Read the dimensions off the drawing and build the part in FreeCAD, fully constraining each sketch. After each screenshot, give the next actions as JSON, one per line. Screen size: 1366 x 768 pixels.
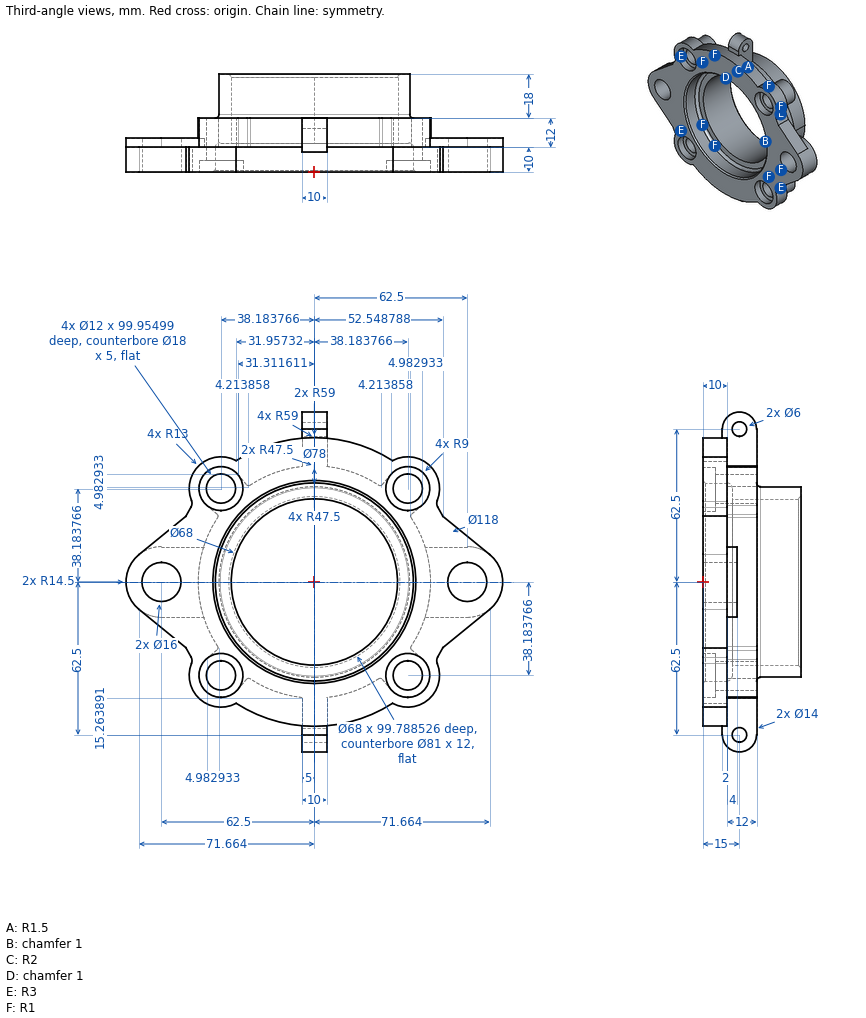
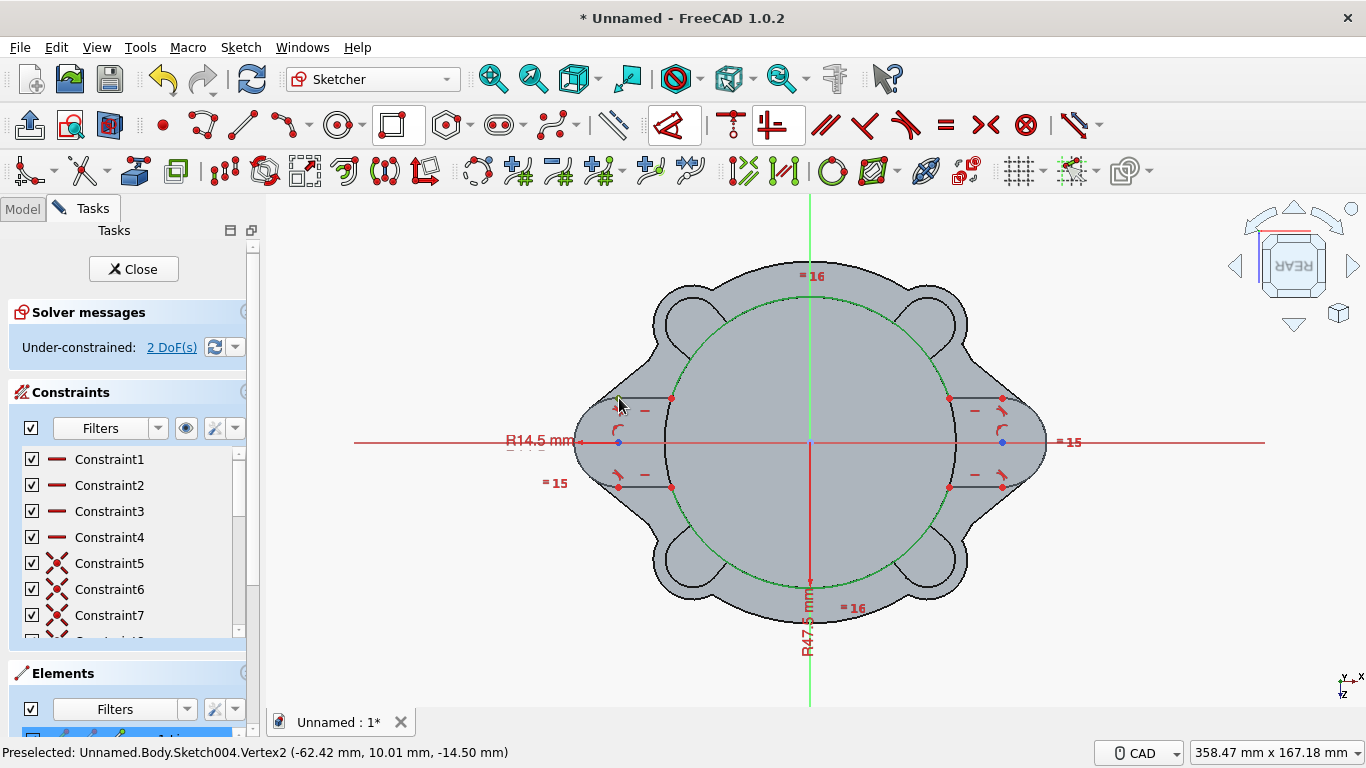
{"action": "key", "text": "l"}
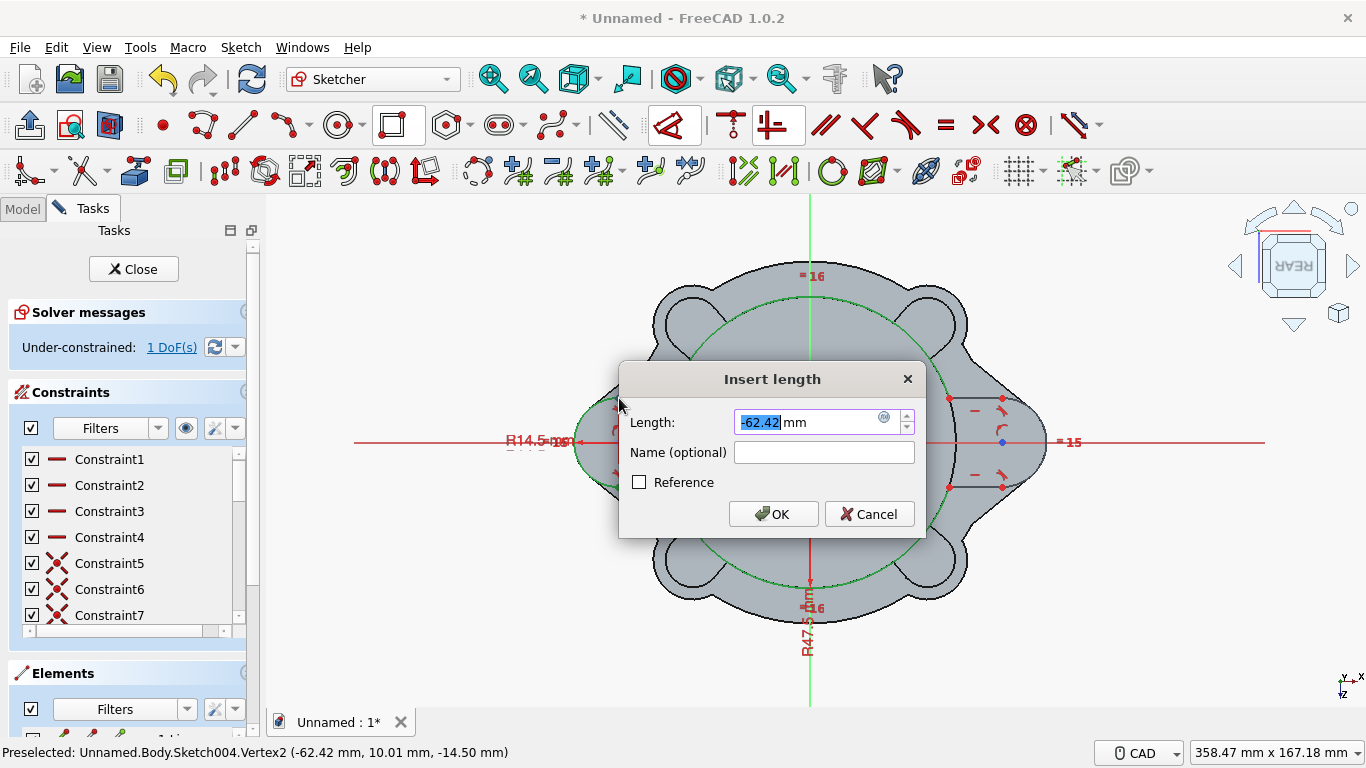
{"action": "type", "text": "-62.5"}
{"action": "key", "text": "Return"}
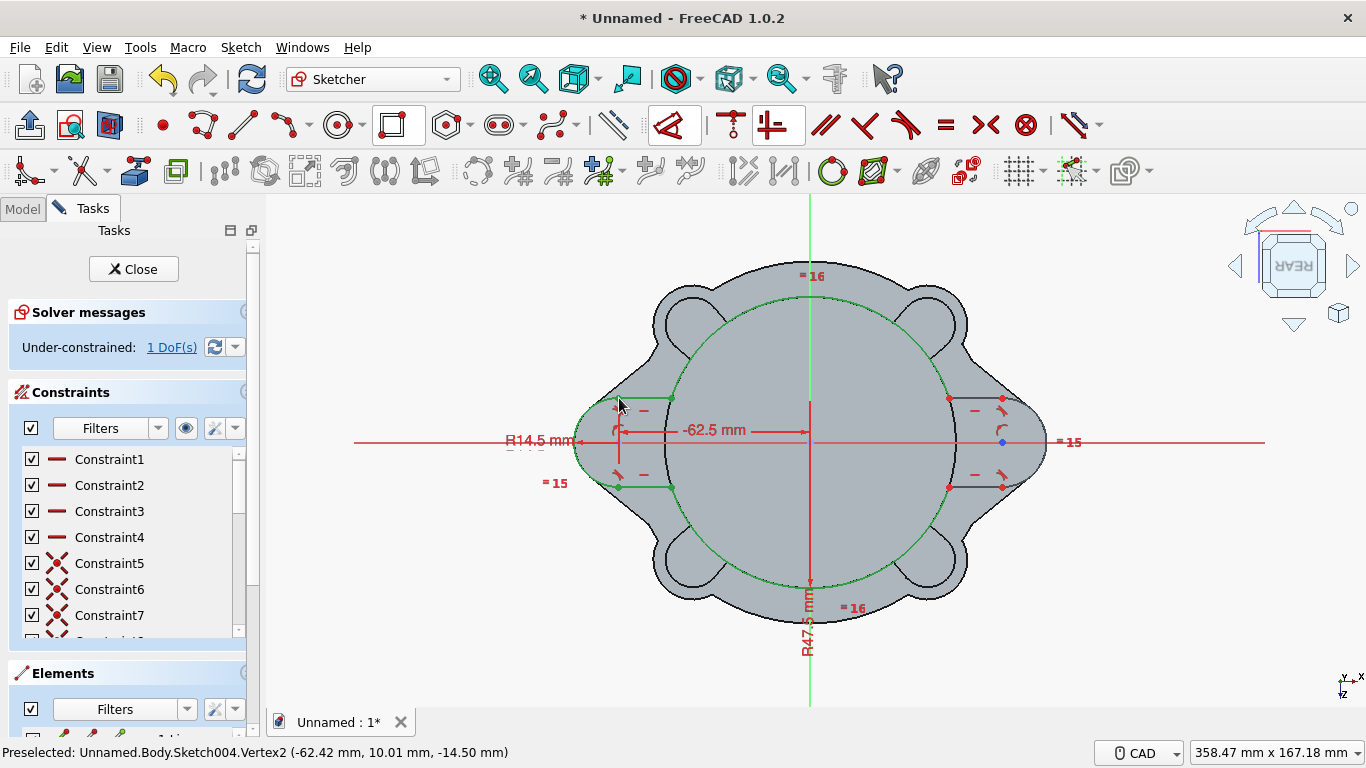
{"action": "left_click", "coordinate": [1002, 487]}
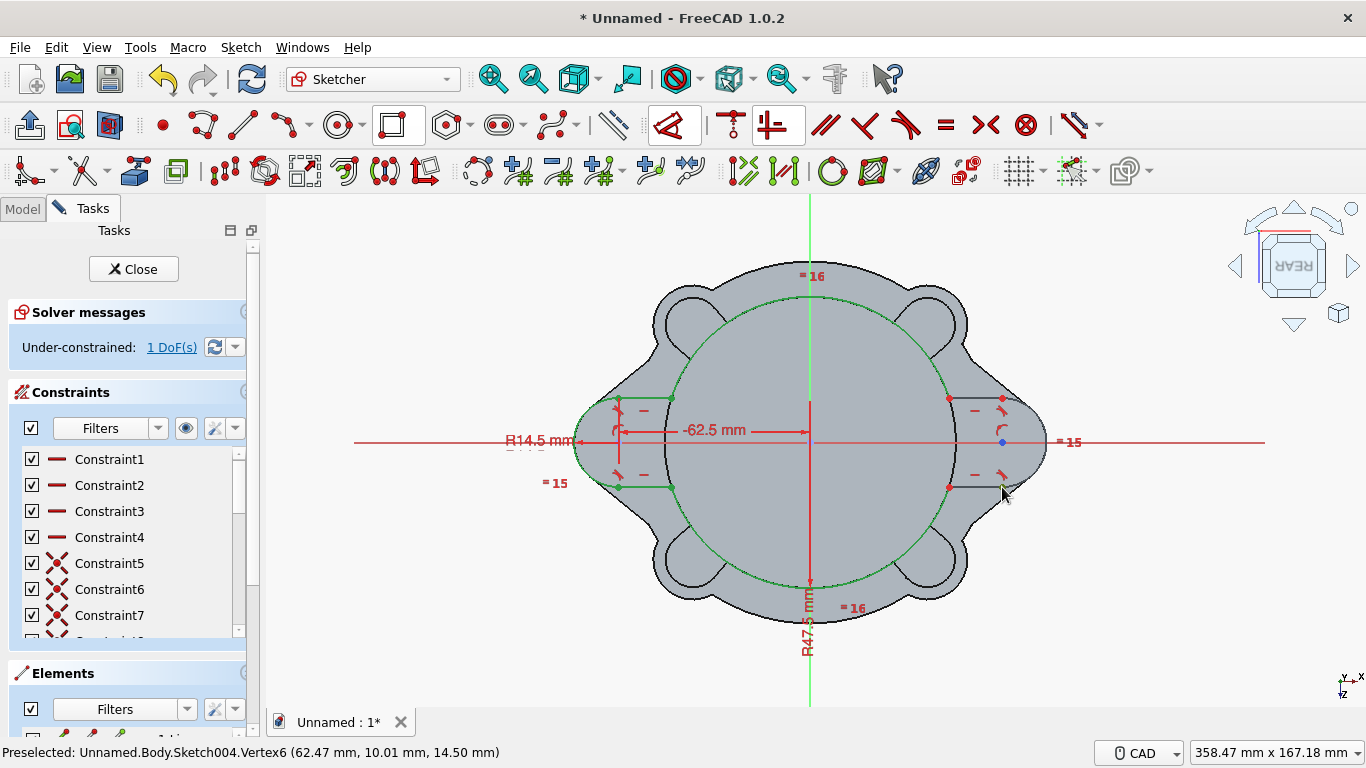
{"action": "left_click", "coordinate": [696, 126]}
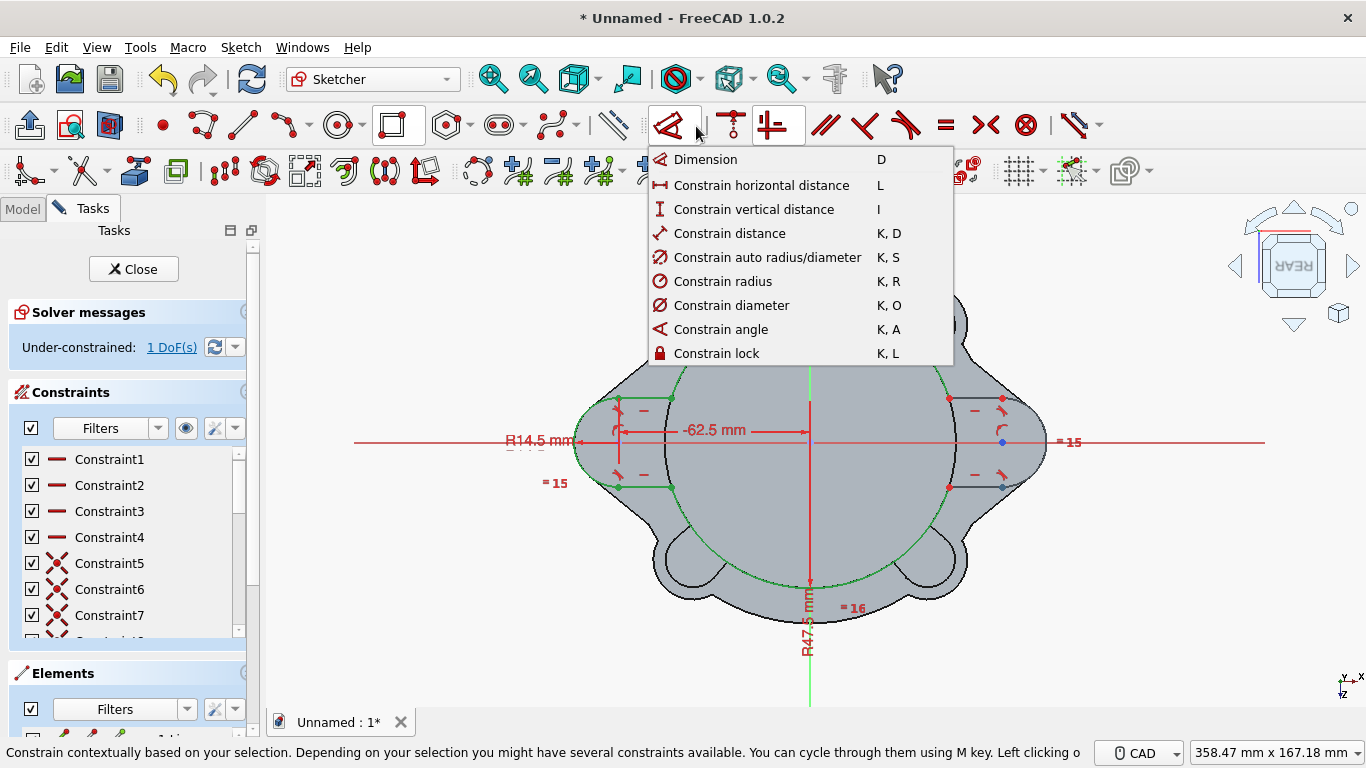
{"action": "left_click", "coordinate": [801, 185]}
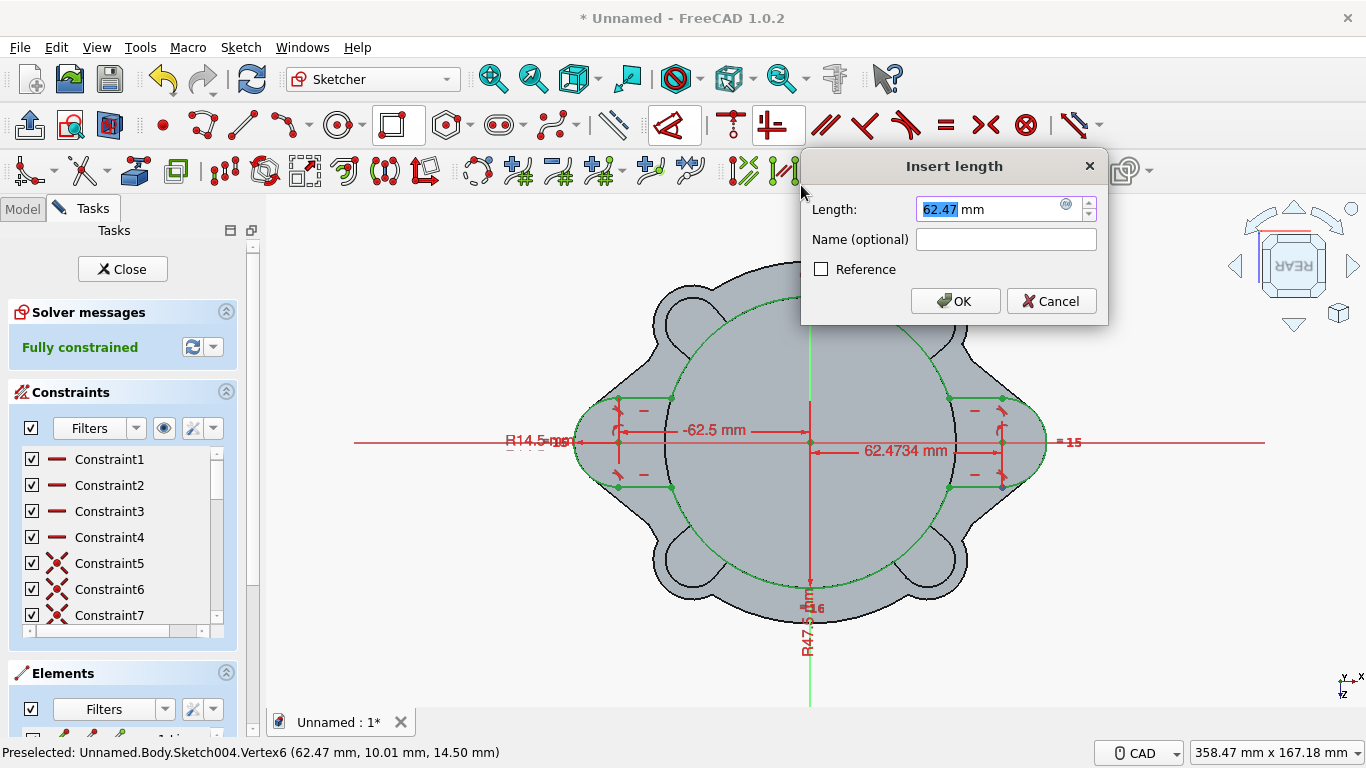
{"action": "type", "text": "62.5"}
{"action": "key", "text": "Return"}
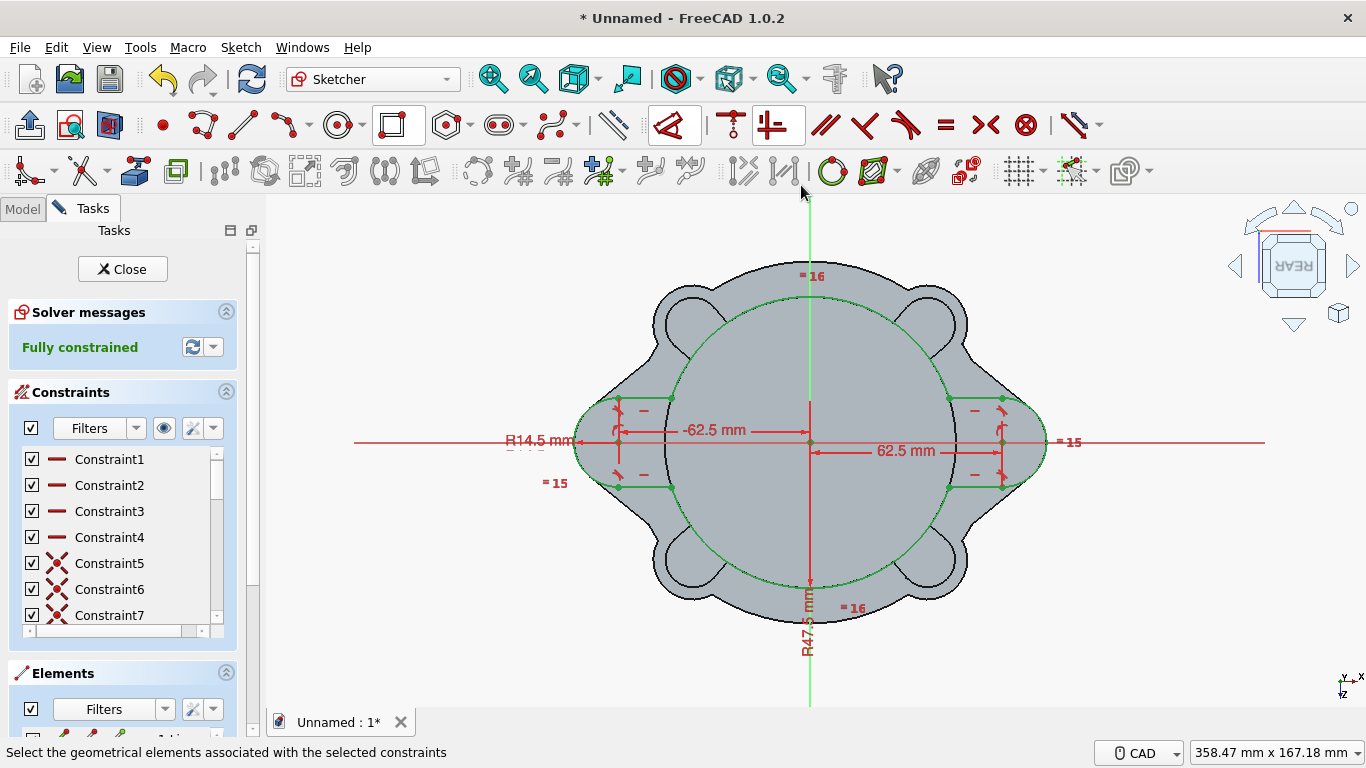
{"action": "left_click", "coordinate": [123, 269]}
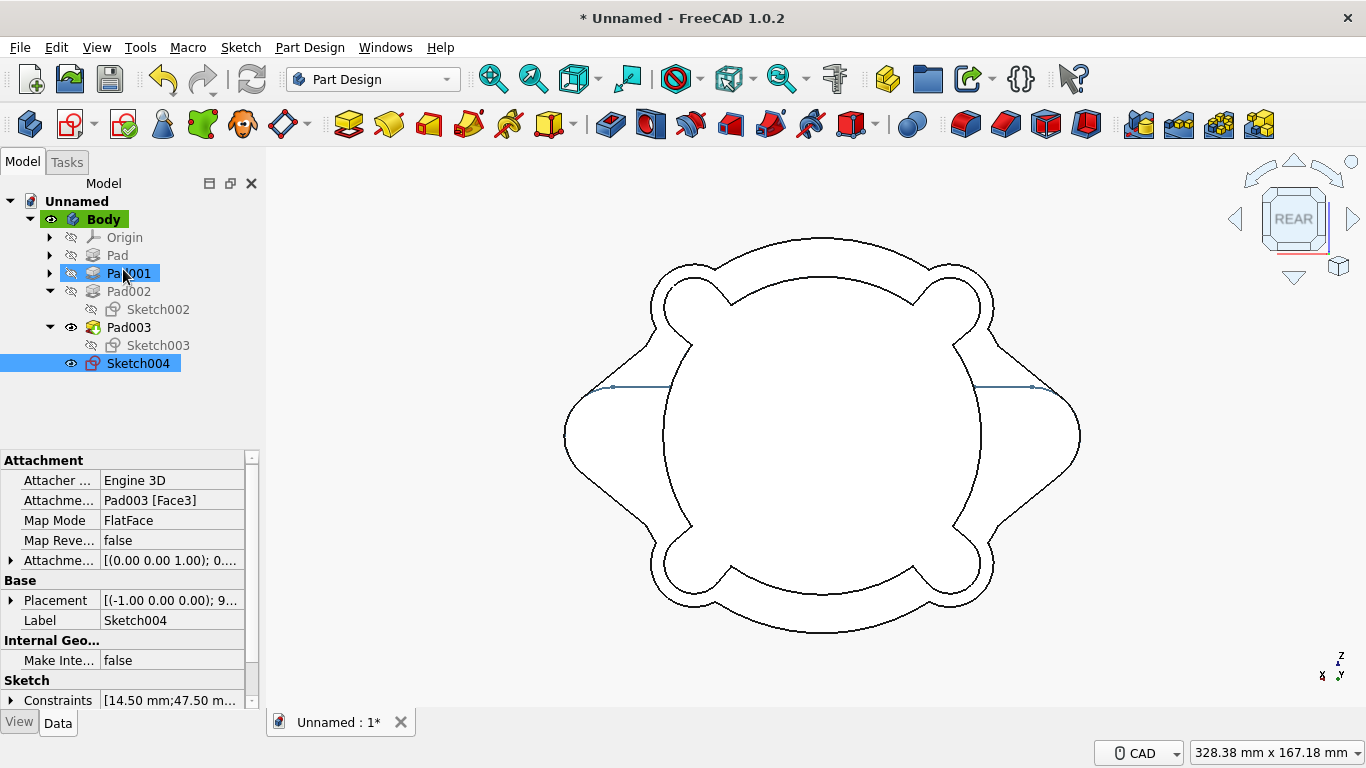
{"action": "left_click", "coordinate": [350, 124]}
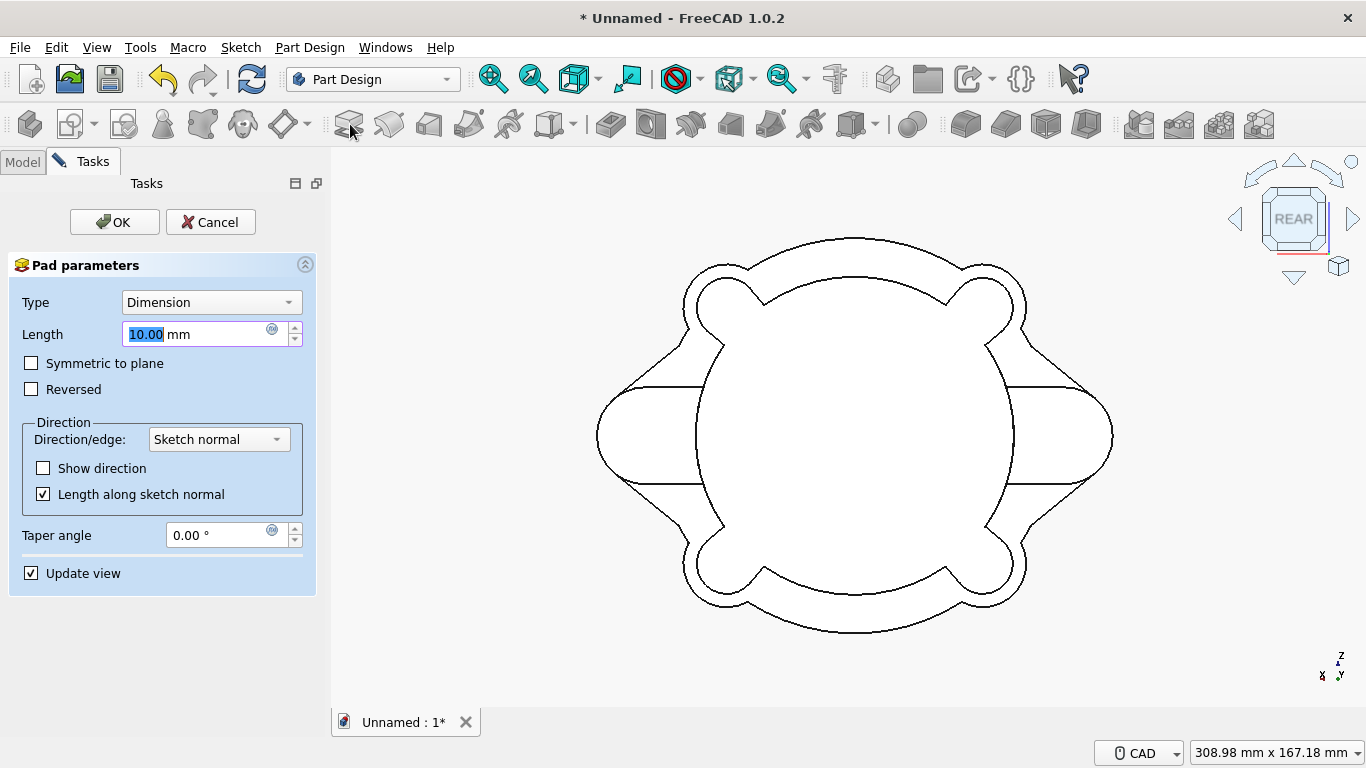
{"action": "type", "text": "4"}
{"action": "key", "text": "Tab"}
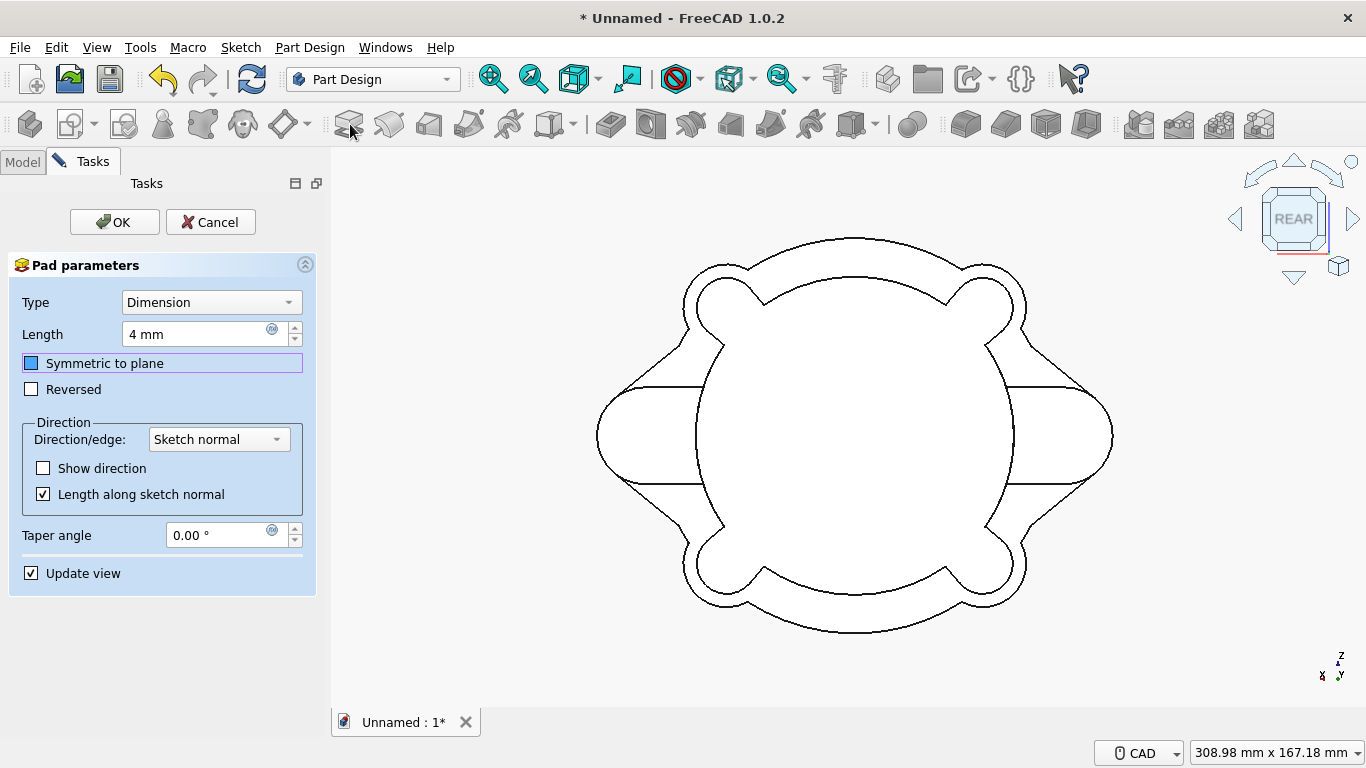
{"action": "left_click", "coordinate": [115, 222]}